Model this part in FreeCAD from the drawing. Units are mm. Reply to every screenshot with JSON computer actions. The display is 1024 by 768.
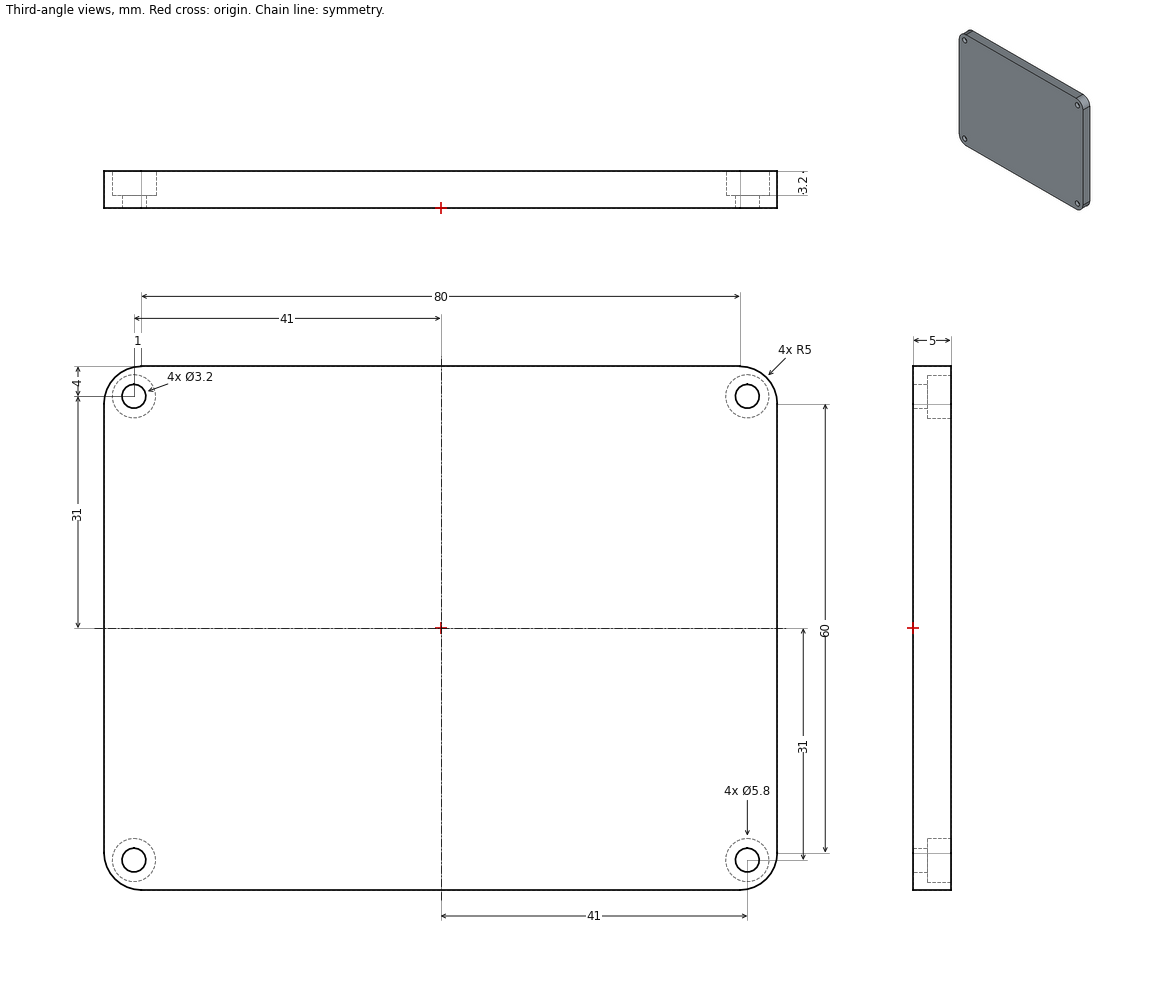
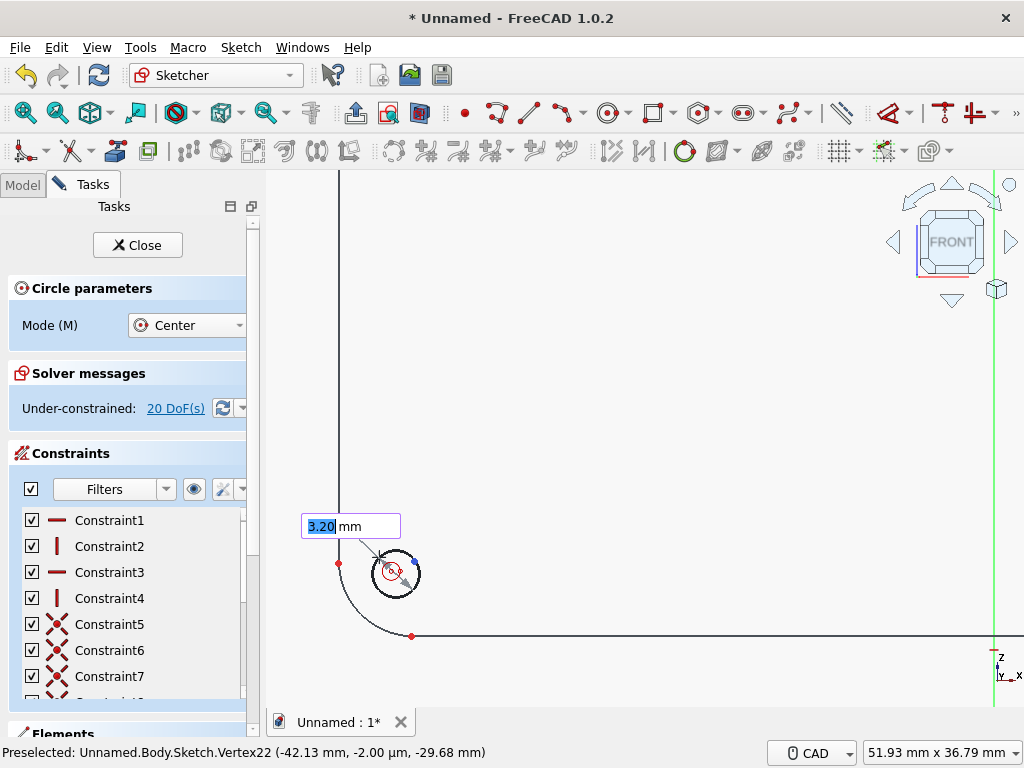
{"action": "type", "text": "3.2"}
{"action": "key", "text": "Return"}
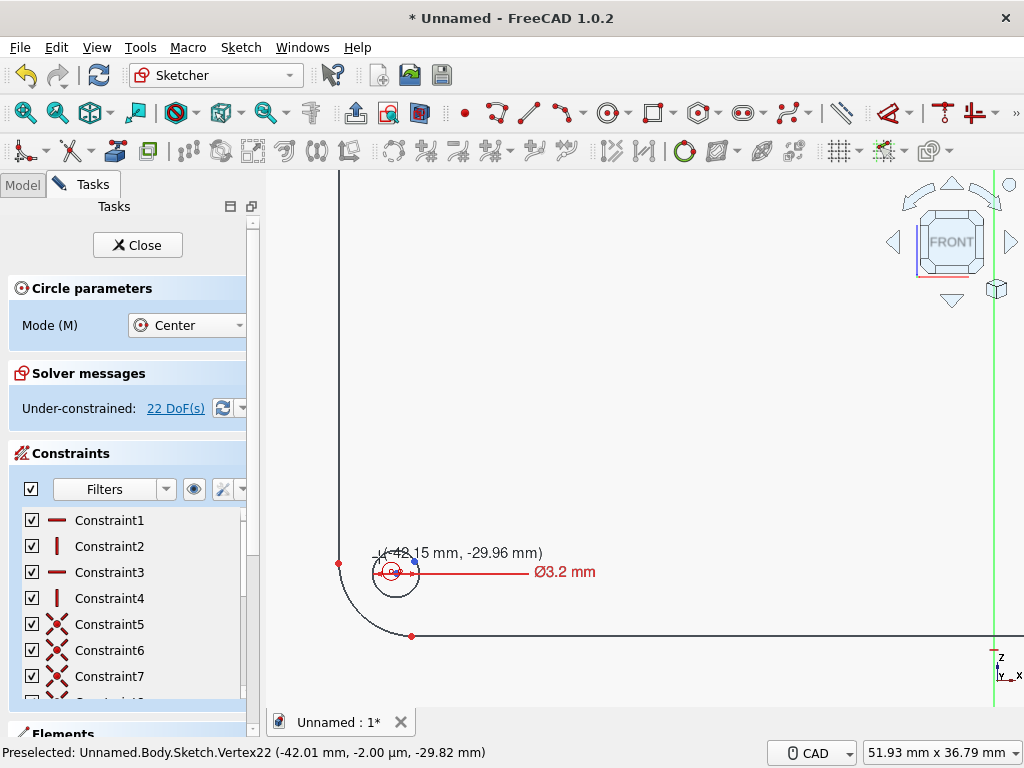
{"action": "scroll", "coordinate": [396, 575], "scroll_direction": "down", "scroll_amount": 6}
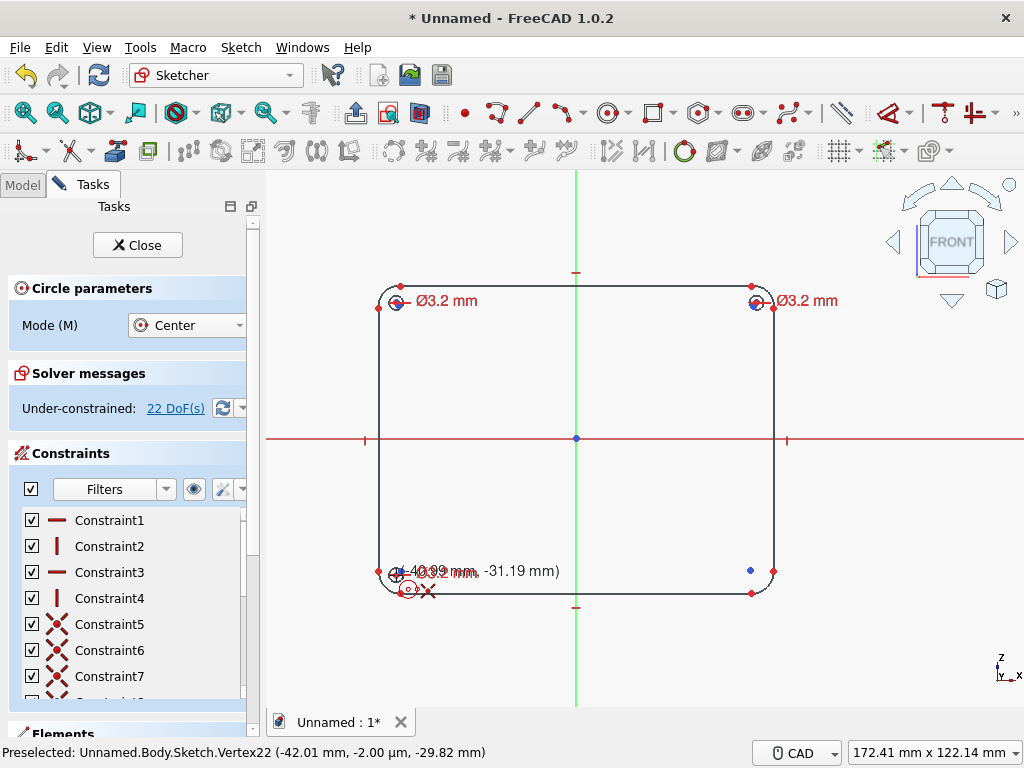
{"action": "scroll", "coordinate": [757, 575], "scroll_direction": "up", "scroll_amount": 6}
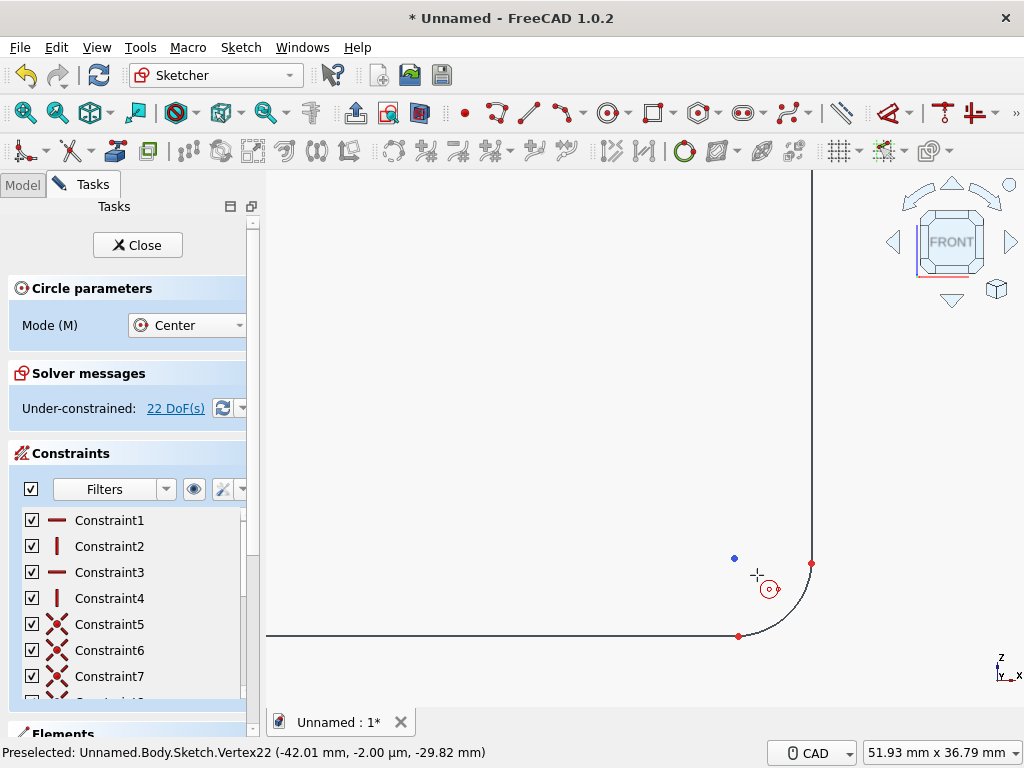
{"action": "left_click", "coordinate": [754, 573]}
{"action": "mouse_move", "coordinate": [771, 557]}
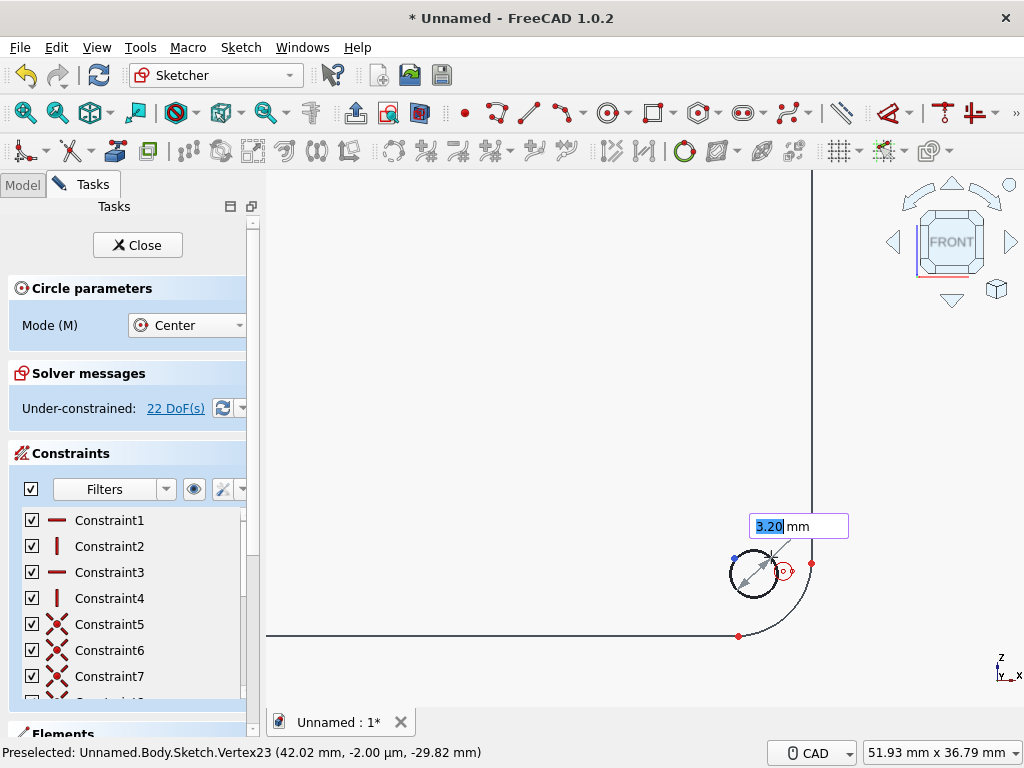
{"action": "type", "text": "3.2"}
{"action": "key", "text": "Return"}
{"action": "key", "text": "Escape"}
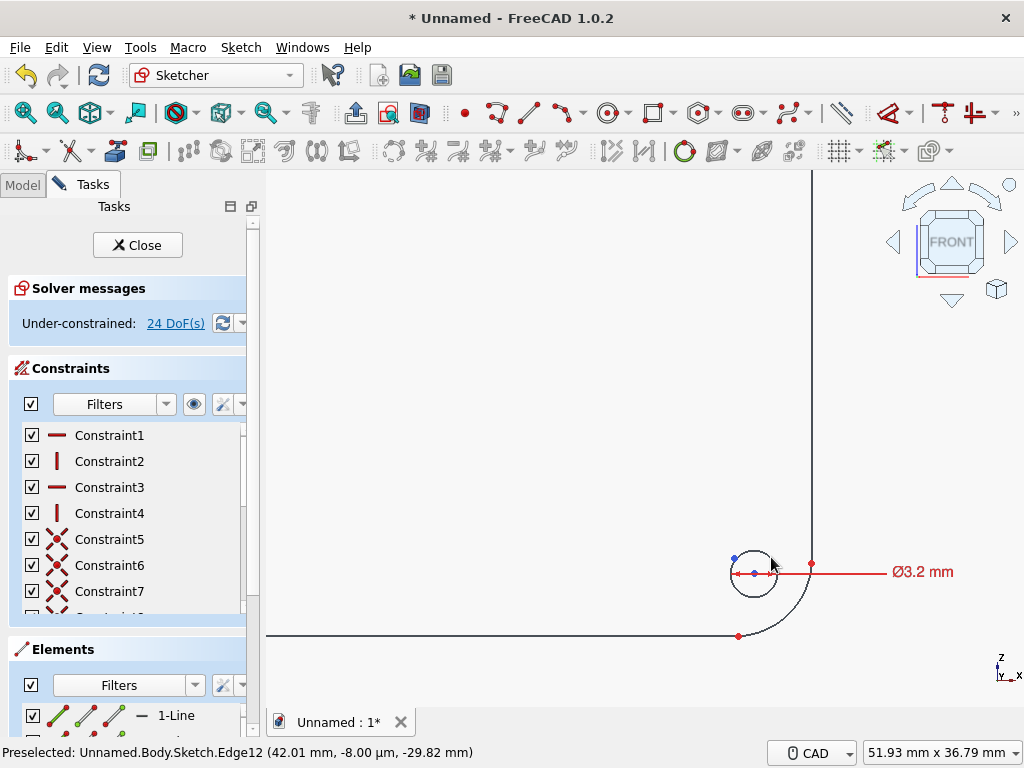
{"action": "scroll", "coordinate": [758, 575], "scroll_direction": "down", "scroll_amount": 6}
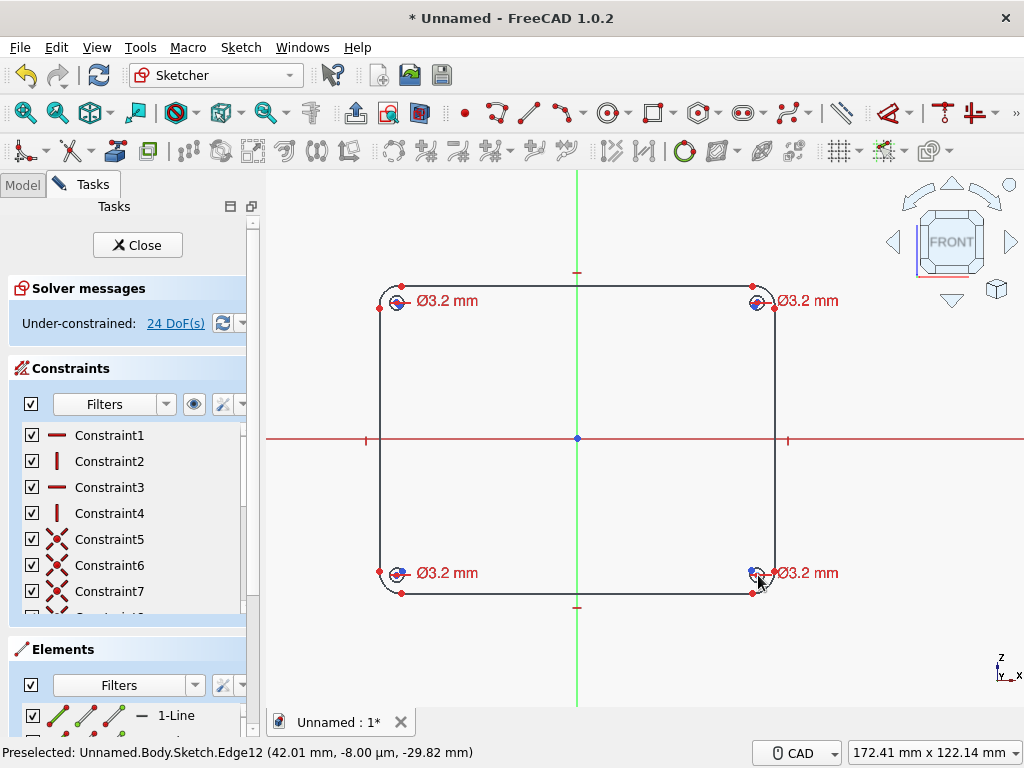
{"action": "left_click", "coordinate": [507, 286]}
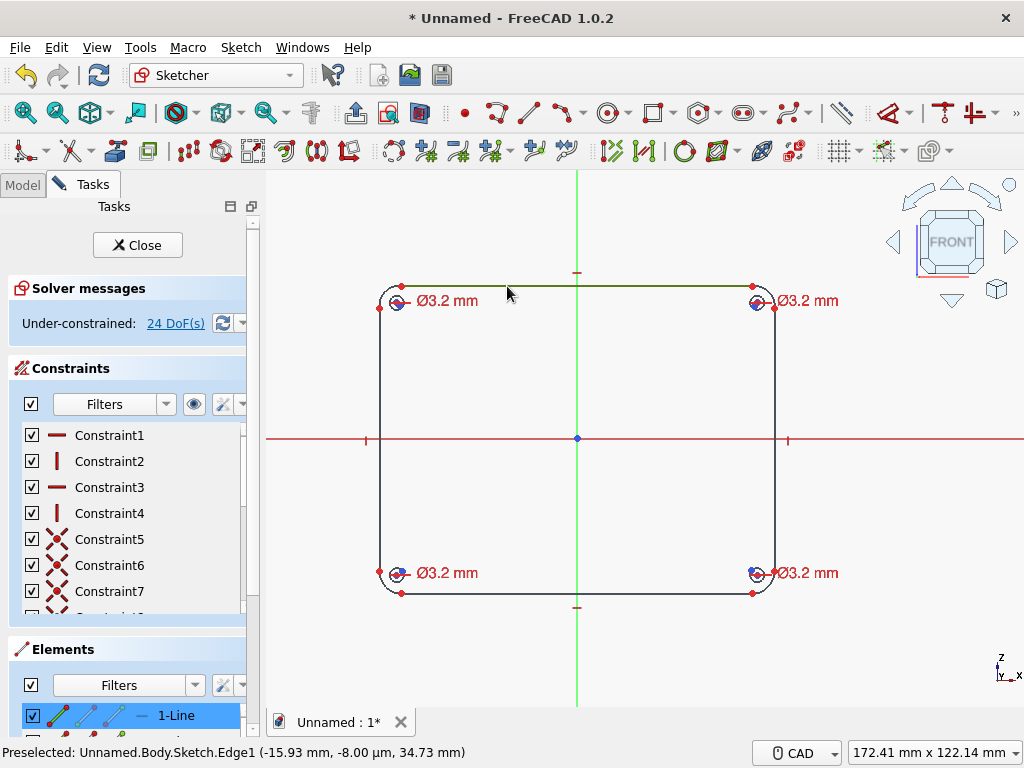
{"action": "scroll", "coordinate": [773, 298], "scroll_direction": "up", "scroll_amount": 2}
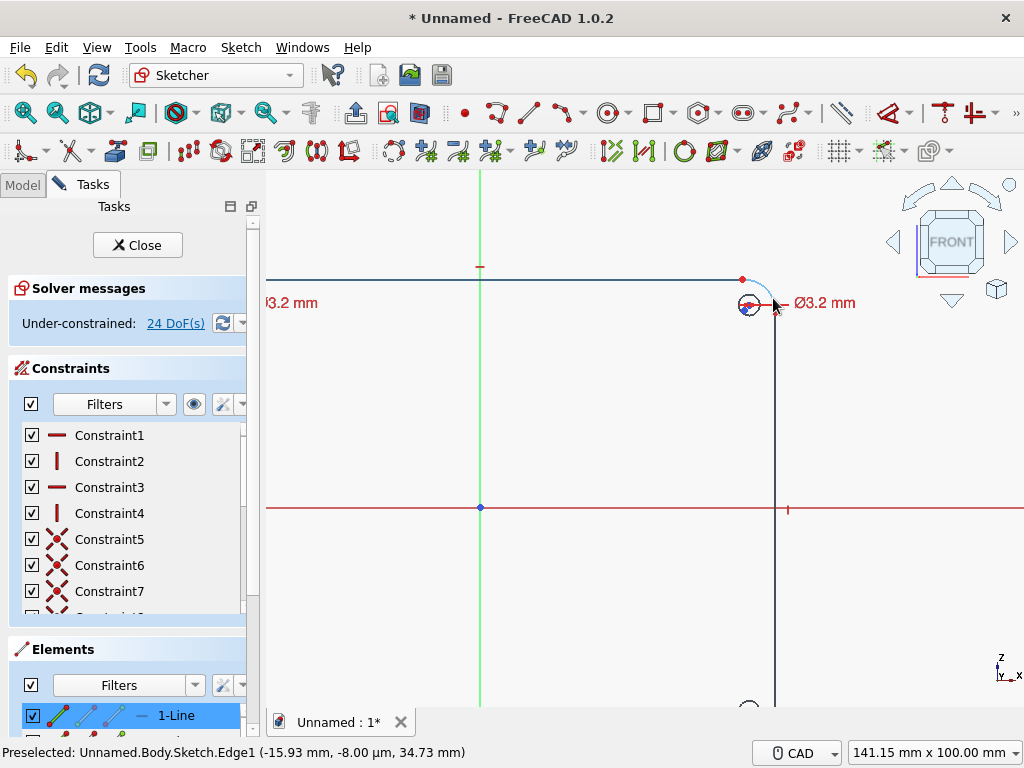
{"action": "left_click", "coordinate": [772, 297]}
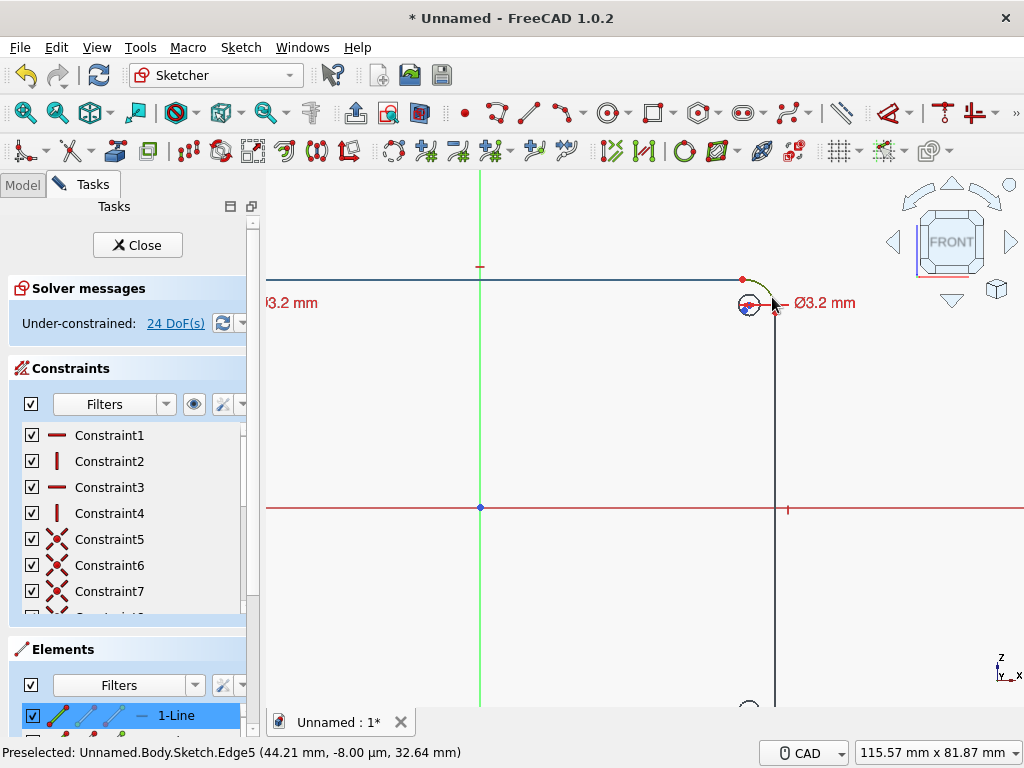
{"action": "key", "text": "t"}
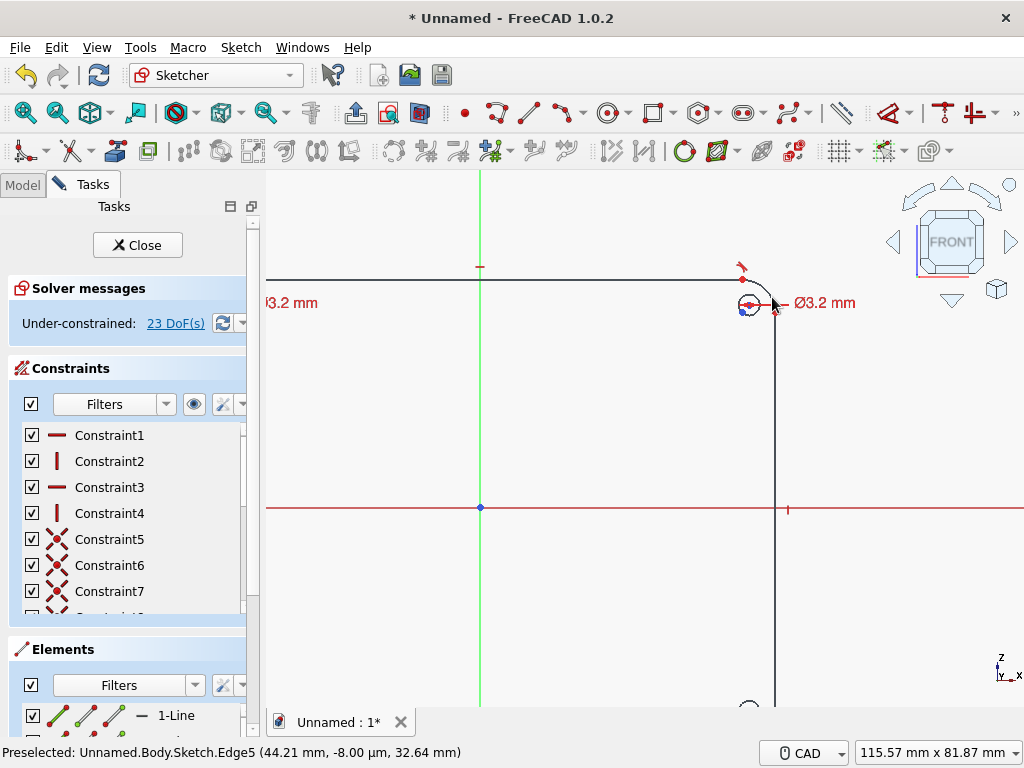
{"action": "left_click", "coordinate": [376, 280]}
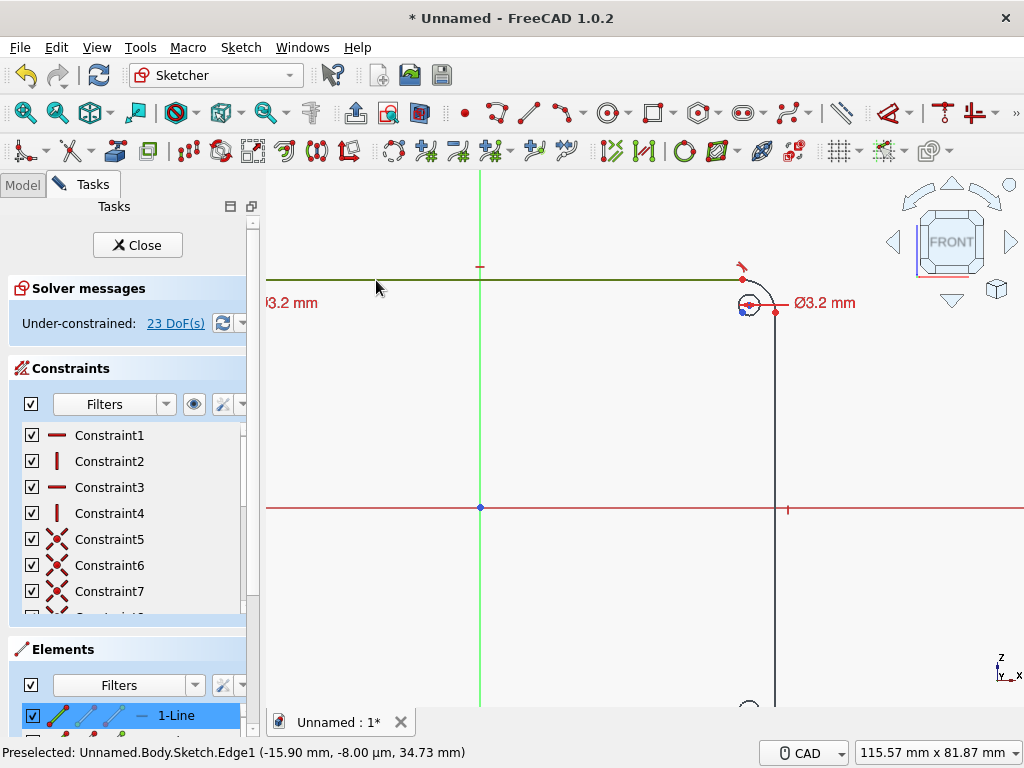
{"action": "scroll", "coordinate": [772, 298], "scroll_direction": "down", "scroll_amount": 2}